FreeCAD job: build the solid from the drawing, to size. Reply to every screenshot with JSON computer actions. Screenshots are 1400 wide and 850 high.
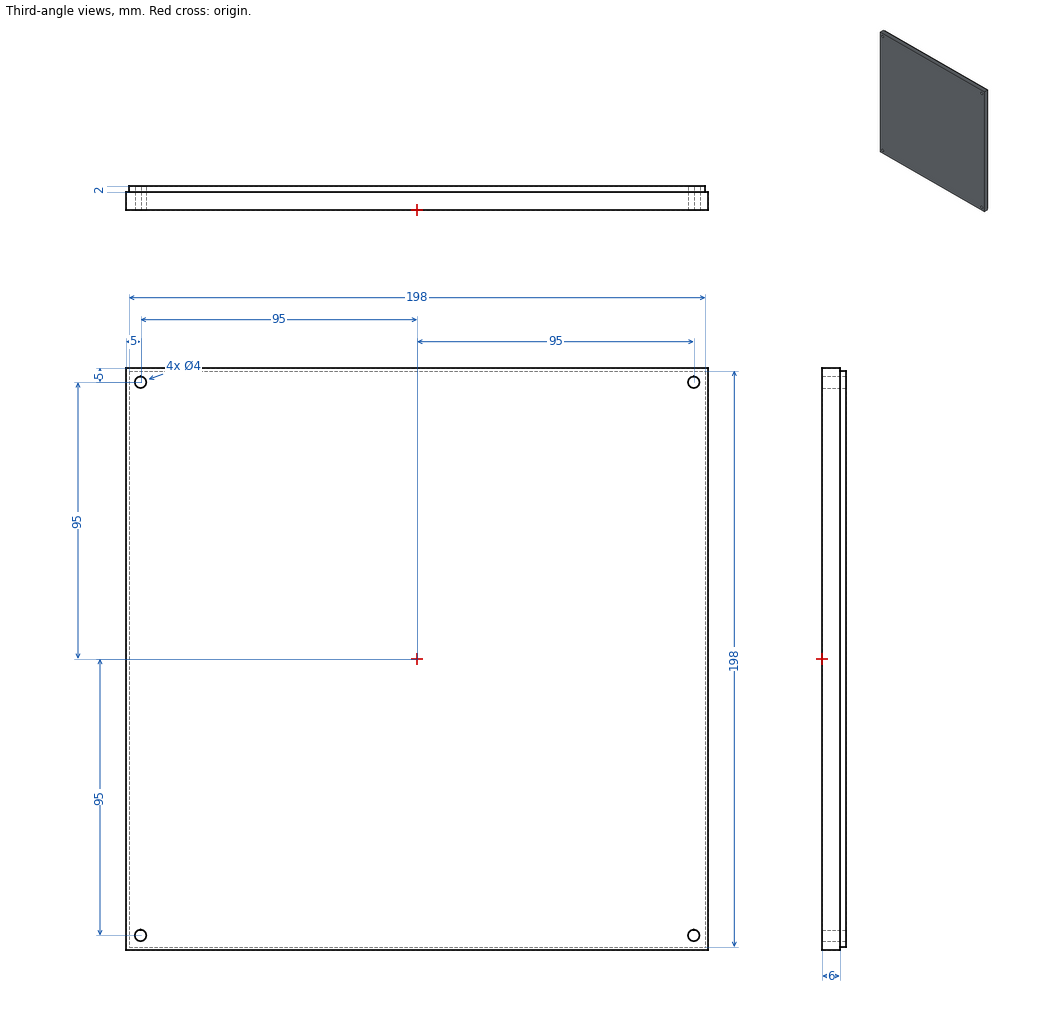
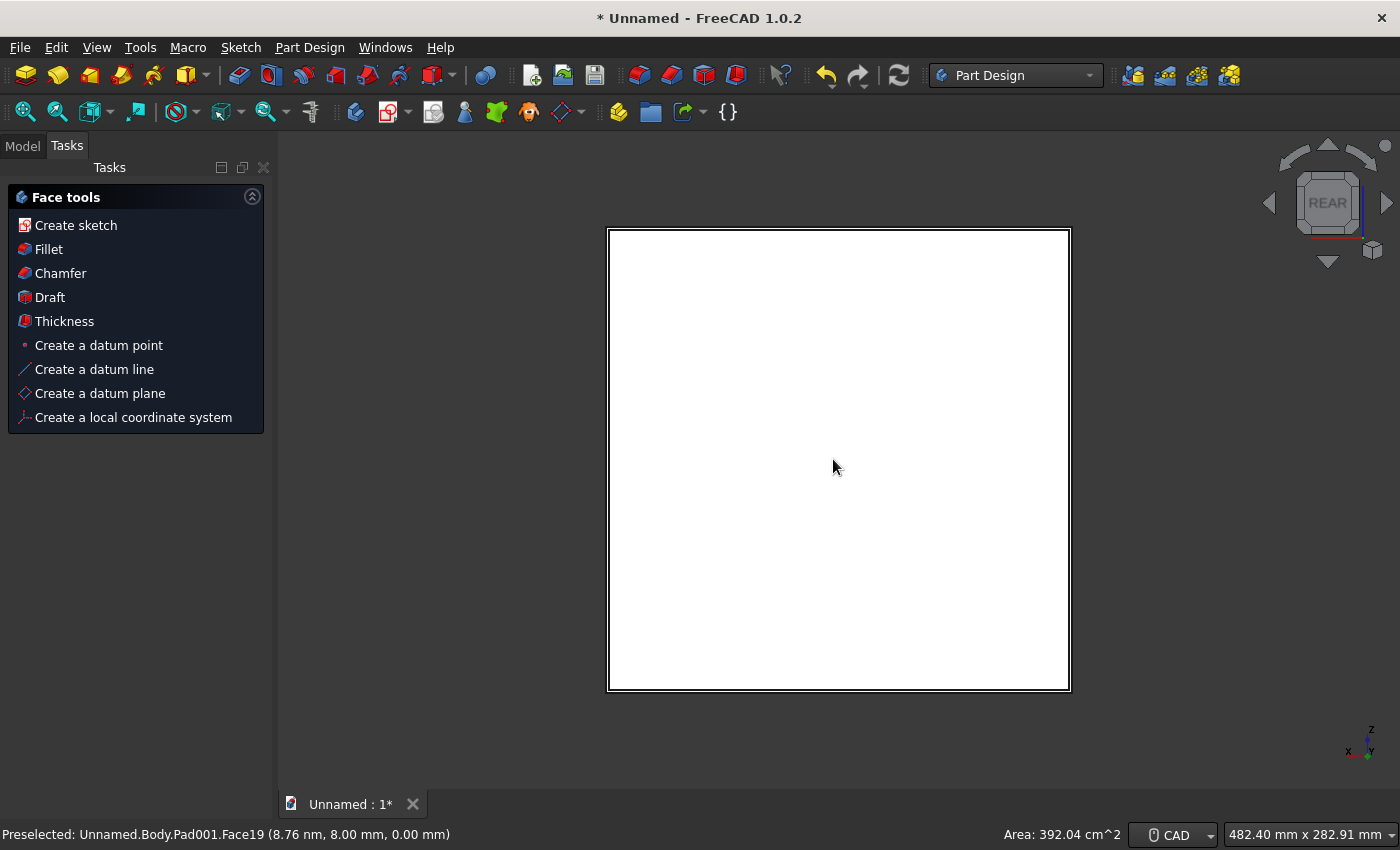
{"action": "left_click", "coordinate": [388, 112]}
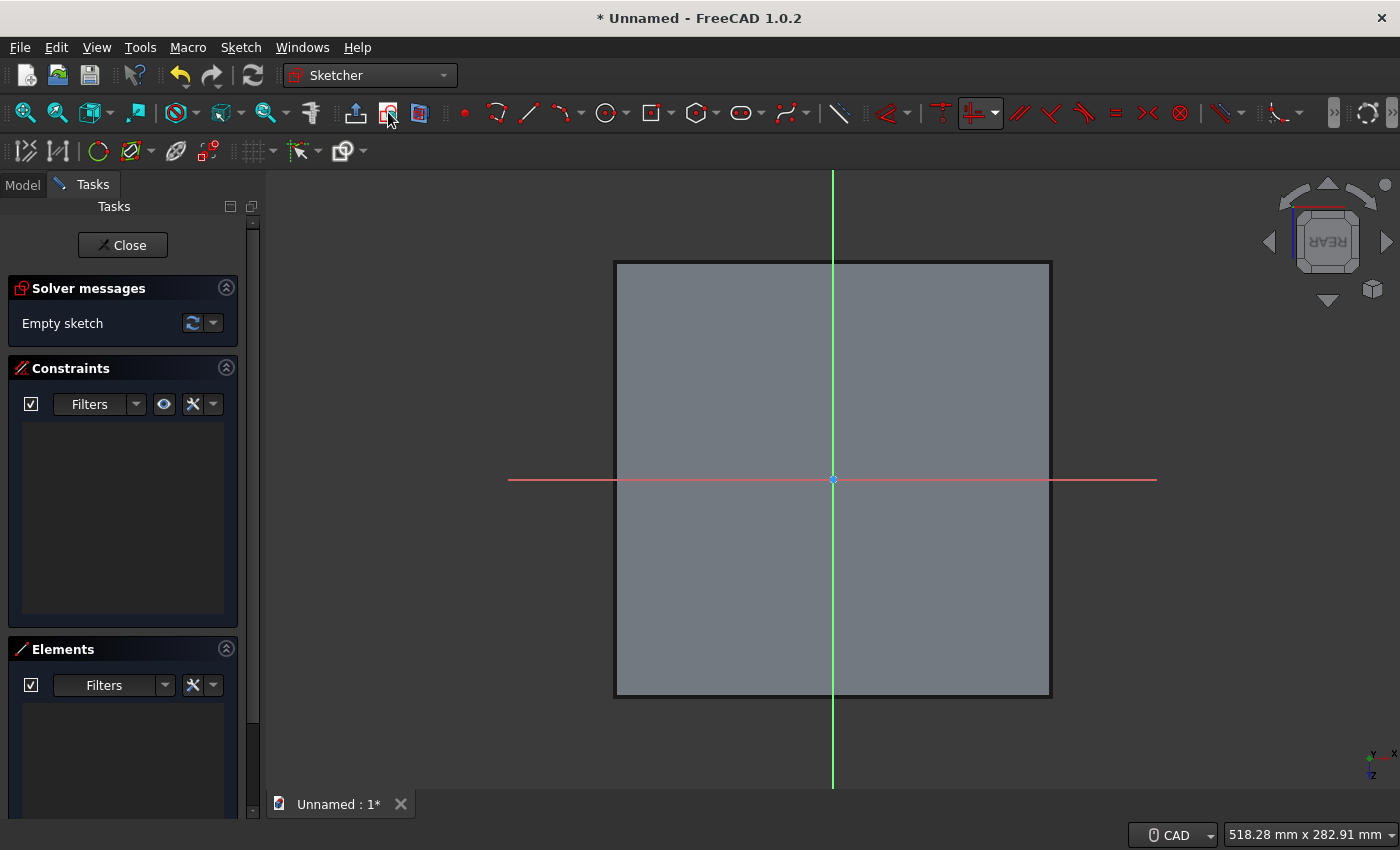
{"action": "left_click", "coordinate": [606, 114]}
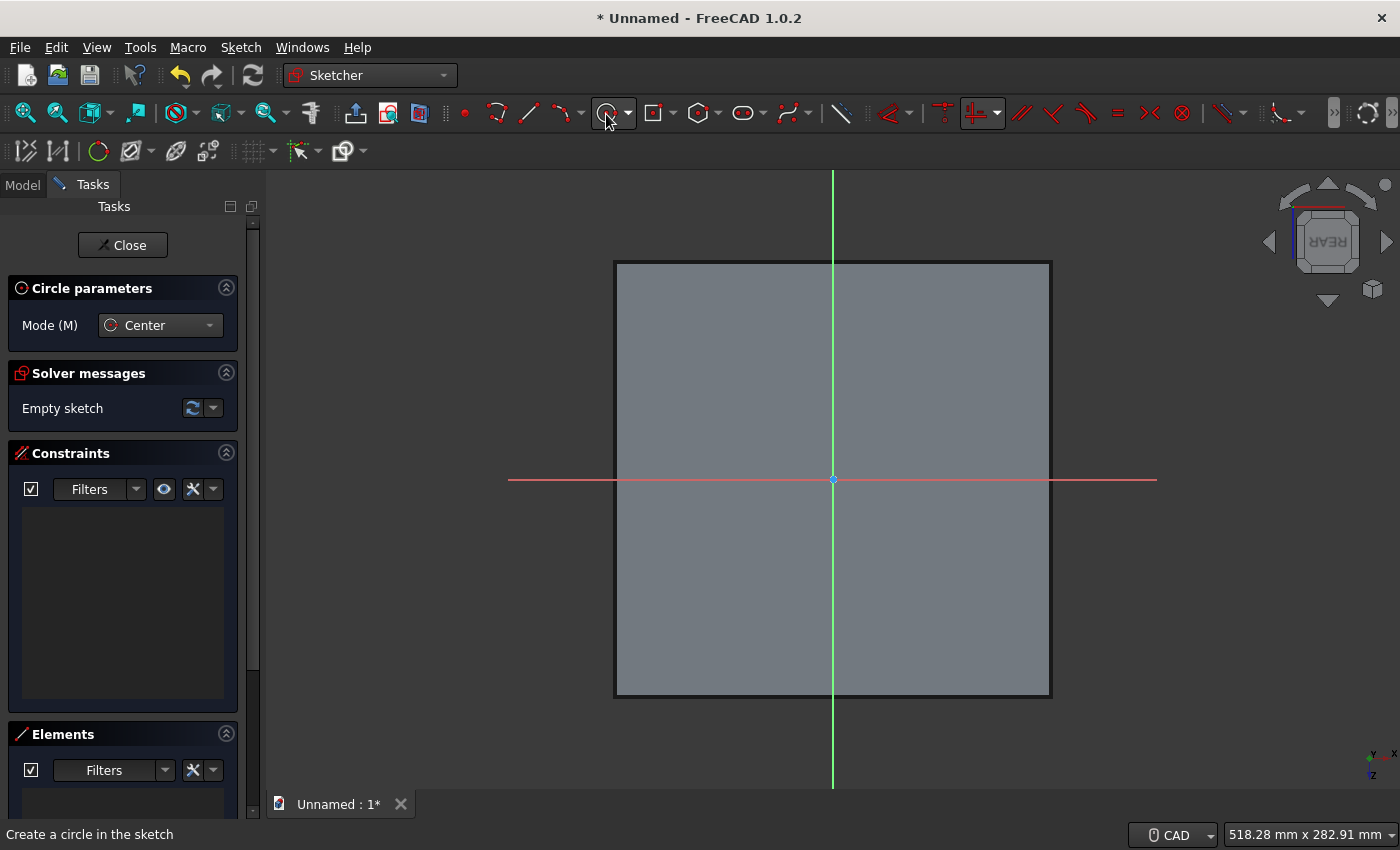
{"action": "scroll", "coordinate": [625, 687], "scroll_direction": "up", "scroll_amount": 9}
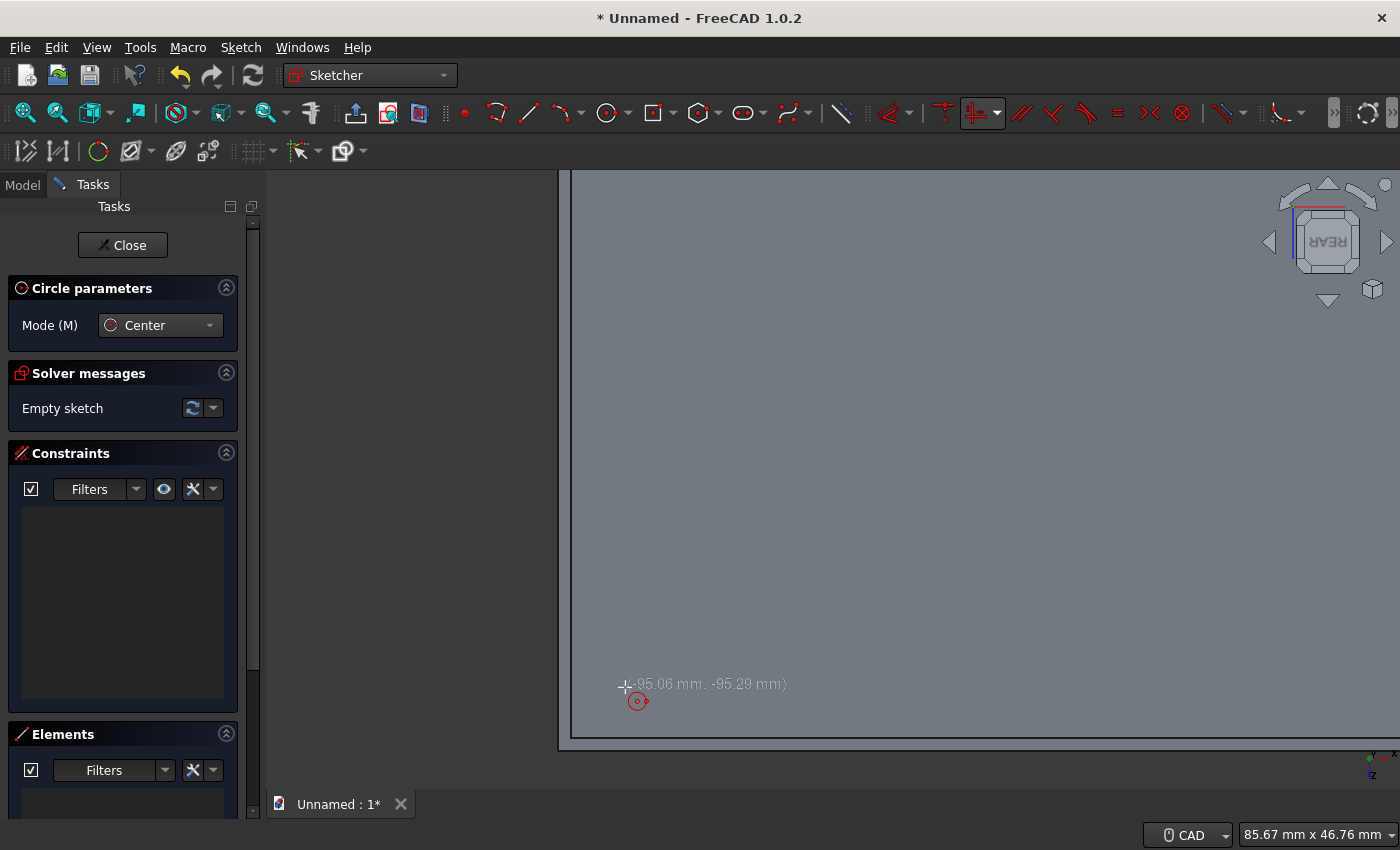
{"action": "scroll", "coordinate": [543, 688], "scroll_direction": "down", "scroll_amount": 9}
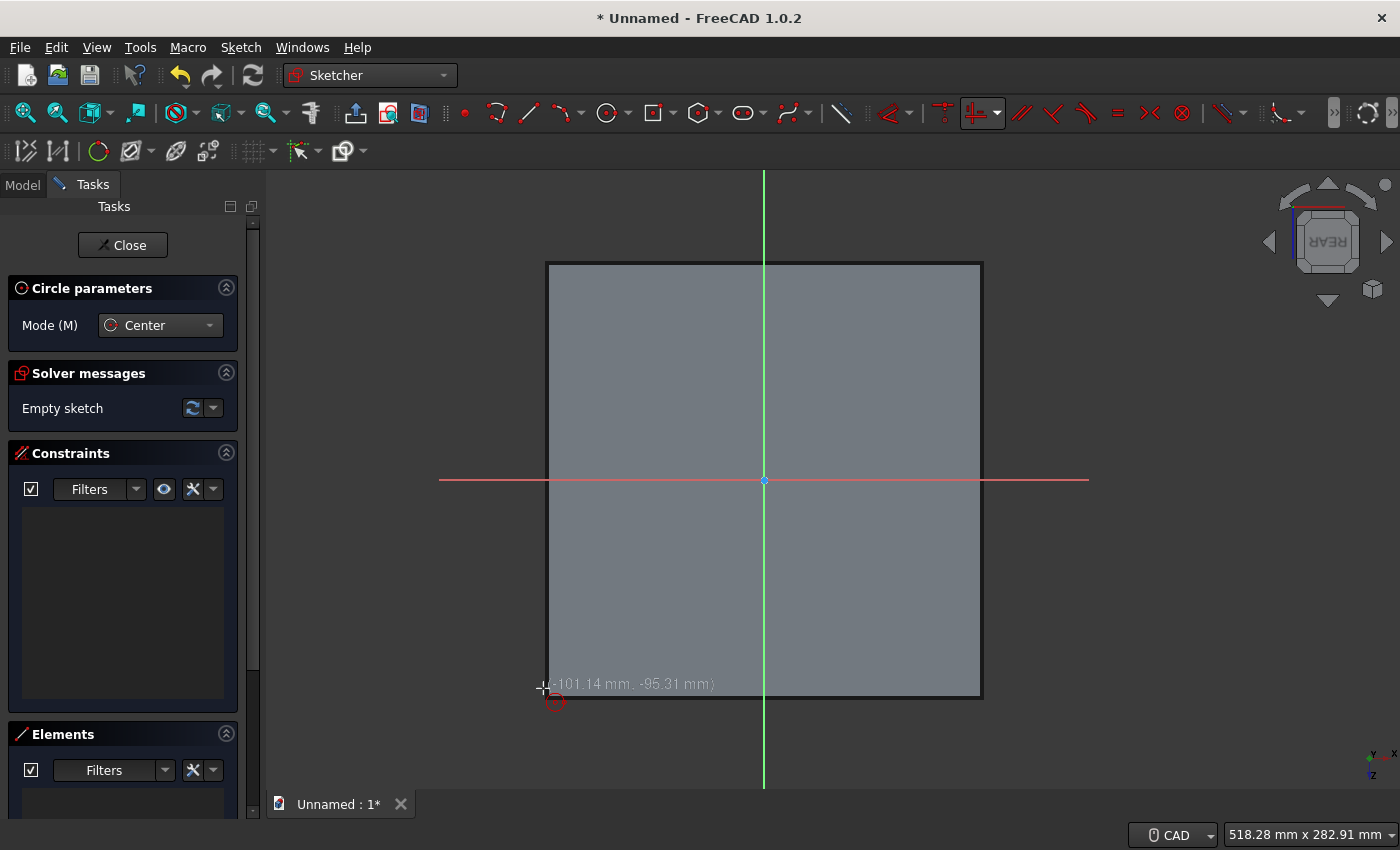
{"action": "left_click", "coordinate": [557, 688]}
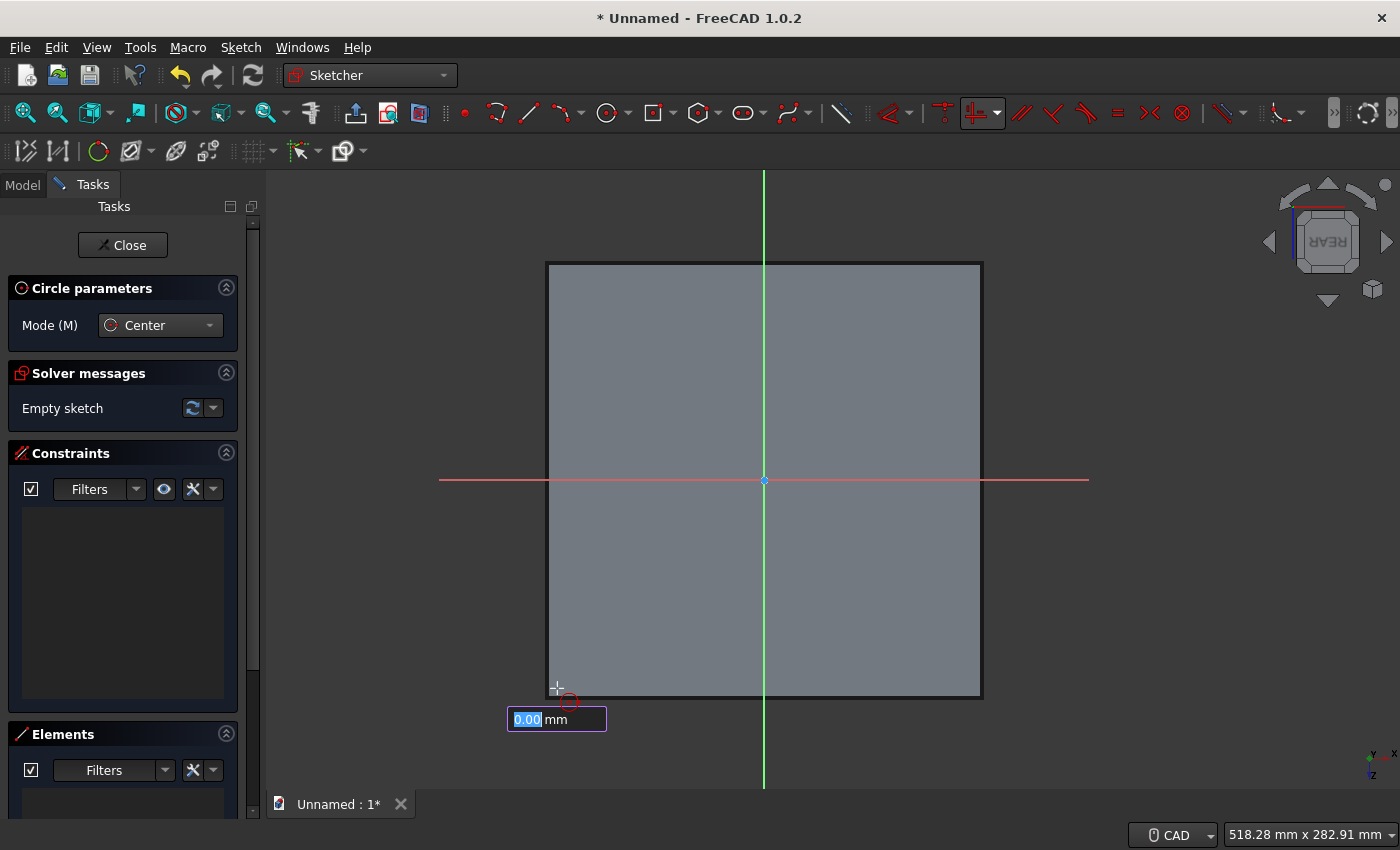
{"action": "scroll", "coordinate": [560, 685], "scroll_direction": "up", "scroll_amount": 7}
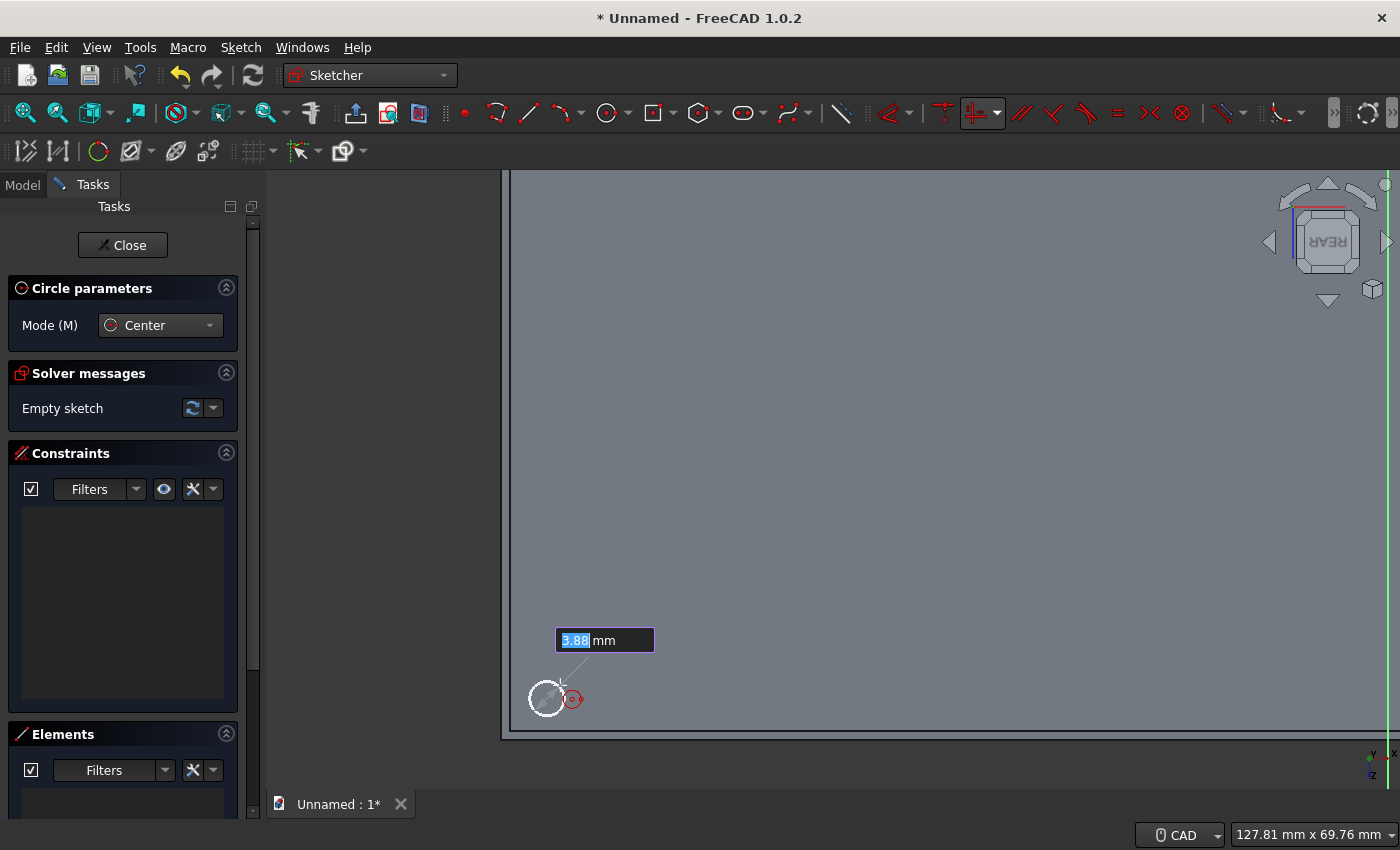
{"action": "left_click", "coordinate": [558, 683]}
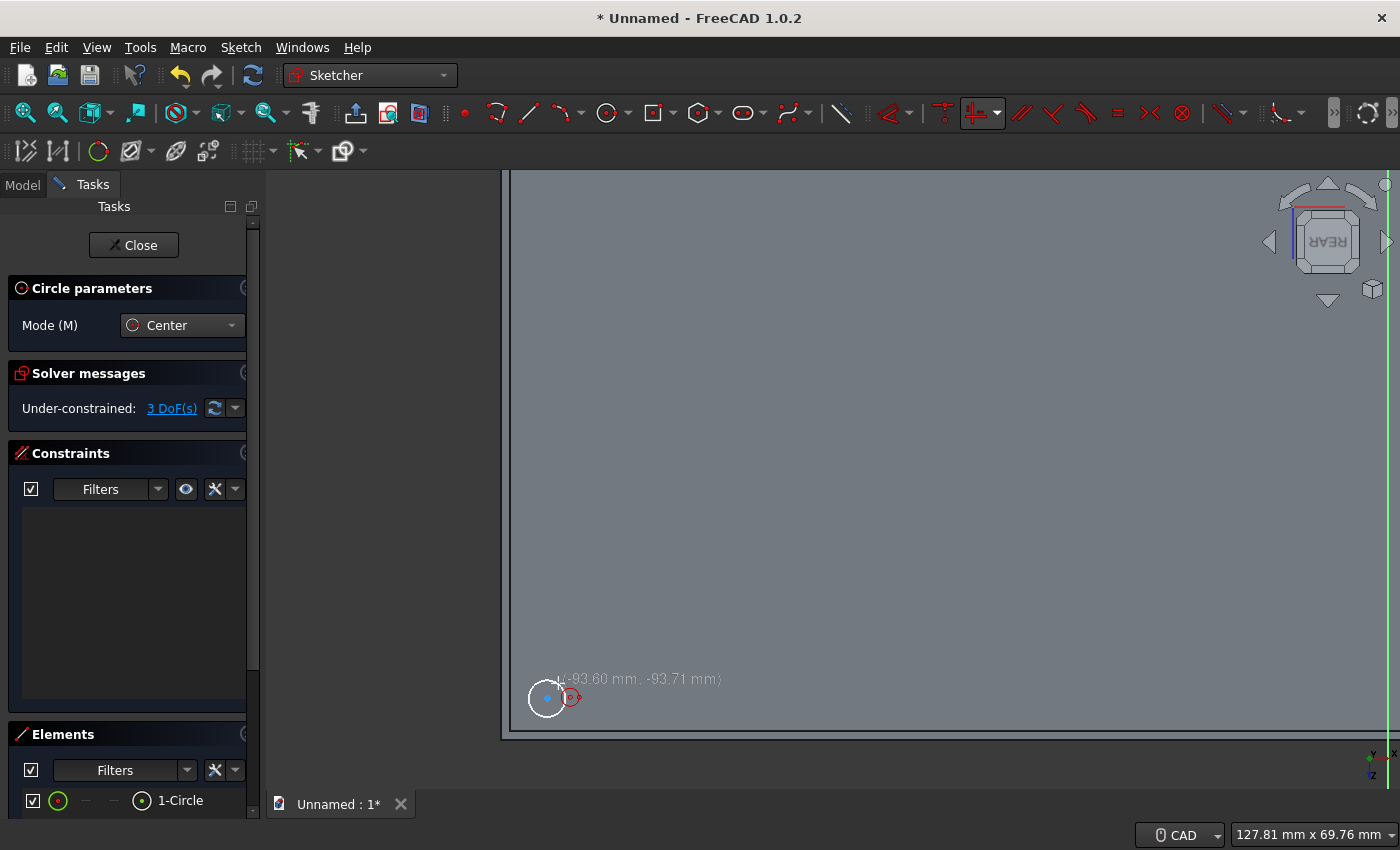
{"action": "scroll", "coordinate": [560, 685], "scroll_direction": "down", "scroll_amount": 7}